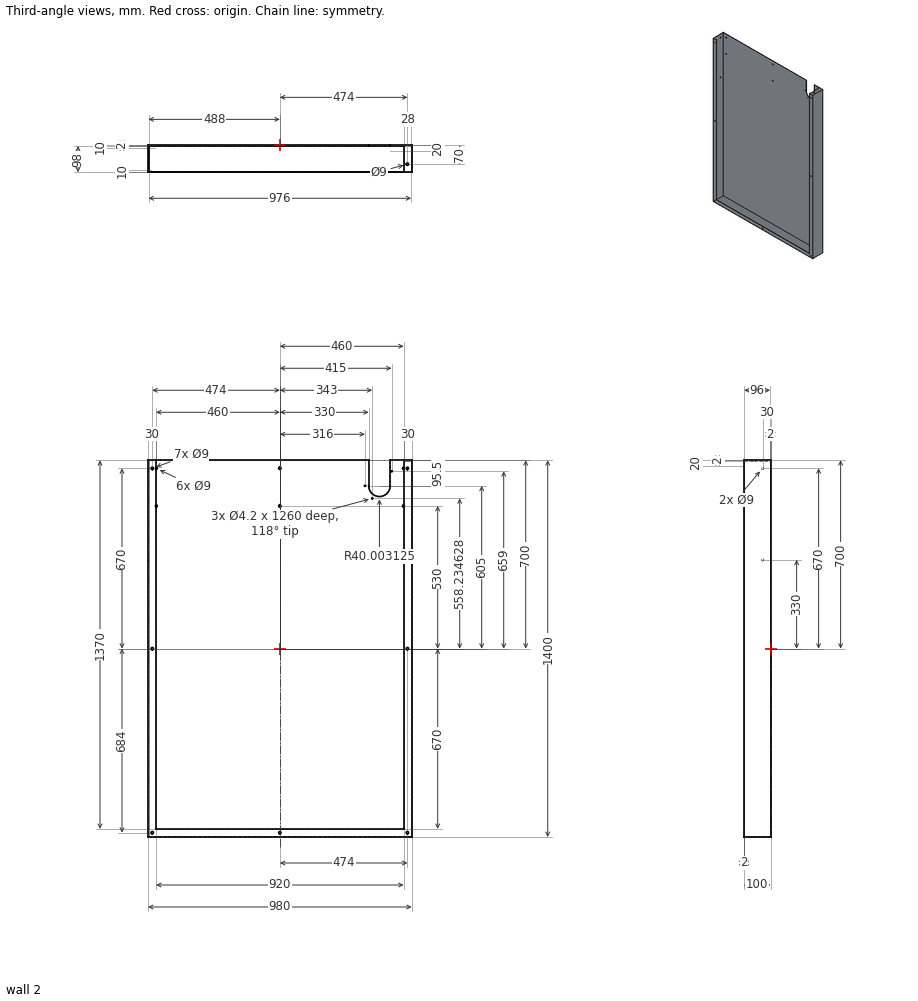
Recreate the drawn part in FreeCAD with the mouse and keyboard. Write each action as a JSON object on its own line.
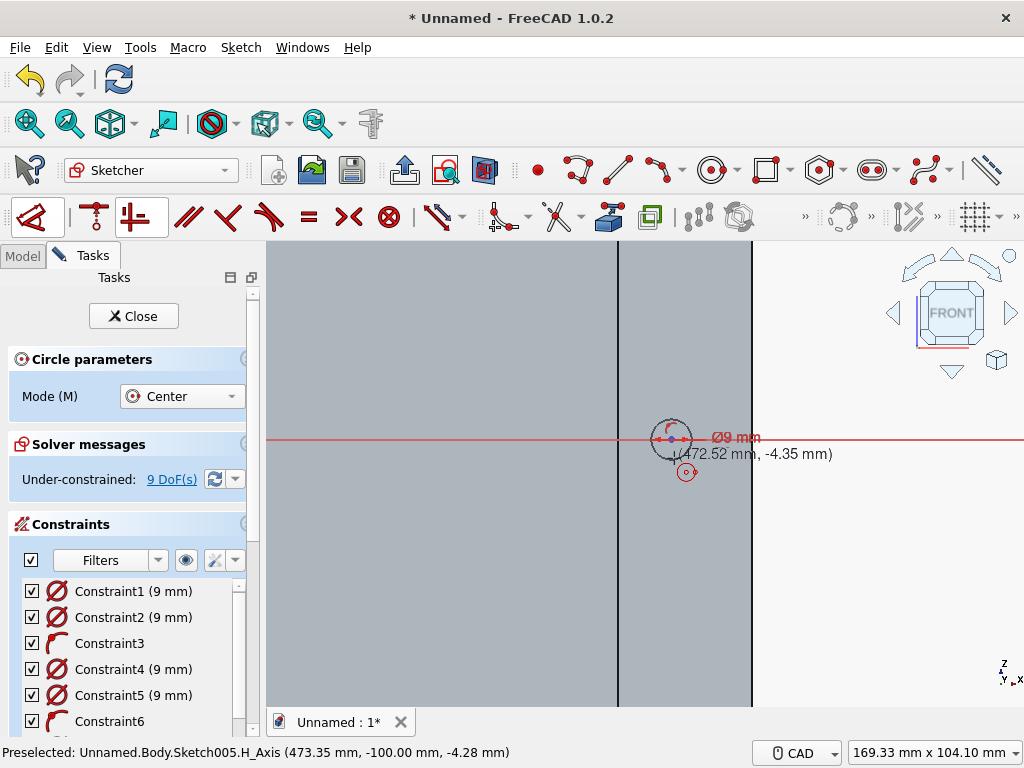
{"action": "scroll", "coordinate": [682, 474], "scroll_direction": "down", "scroll_amount": 15}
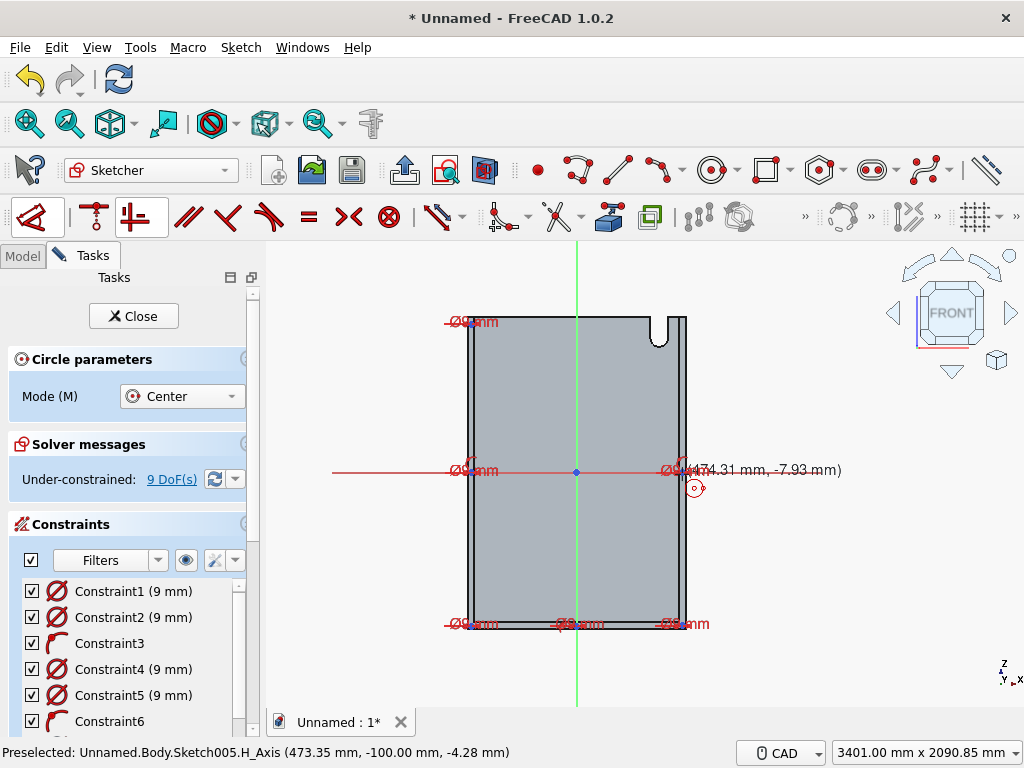
{"action": "scroll", "coordinate": [682, 323], "scroll_direction": "up", "scroll_amount": 16}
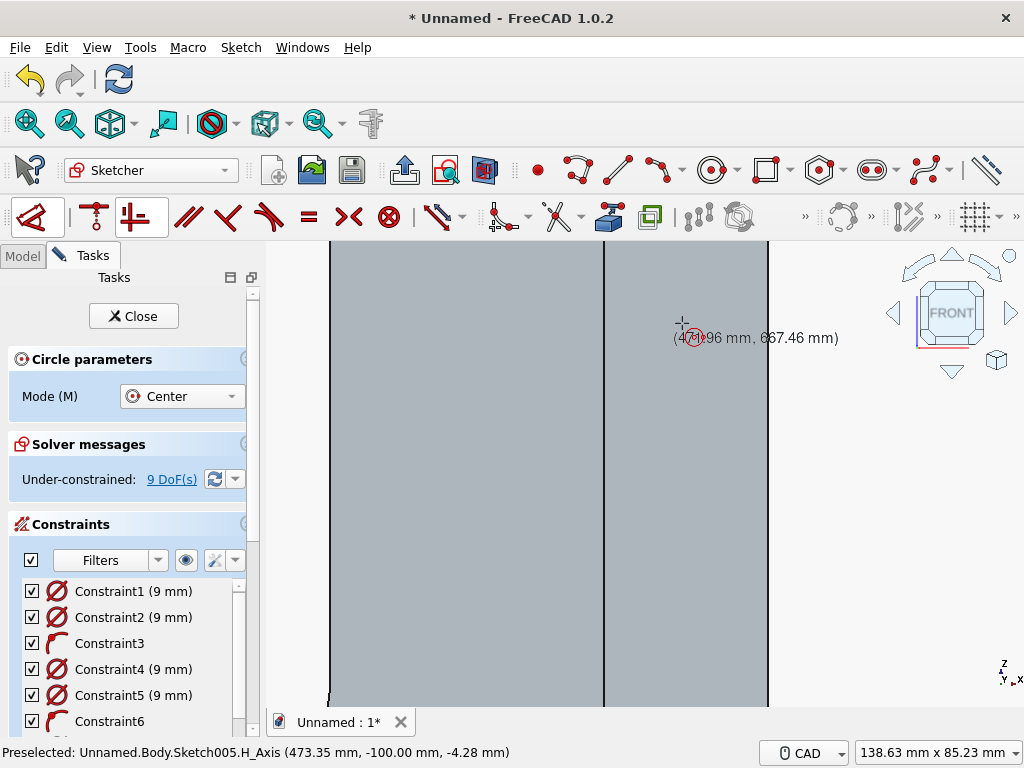
{"action": "scroll", "coordinate": [682, 323], "scroll_direction": "down", "scroll_amount": 16}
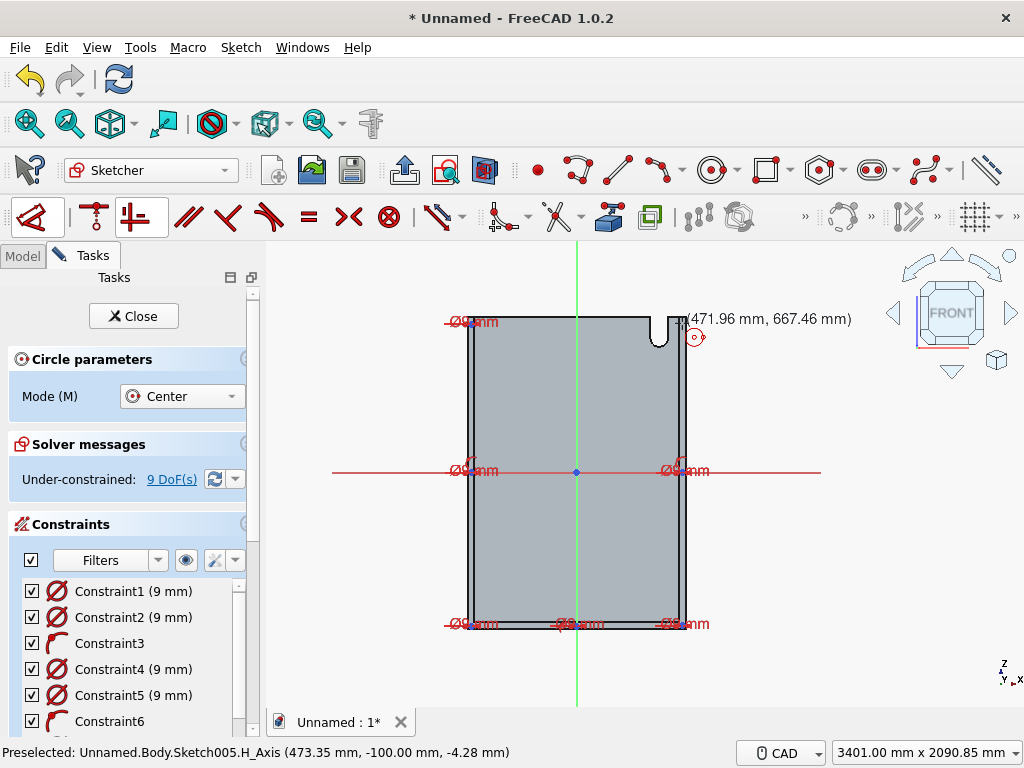
{"action": "left_click", "coordinate": [682, 323]}
{"action": "mouse_move", "coordinate": [683, 323]}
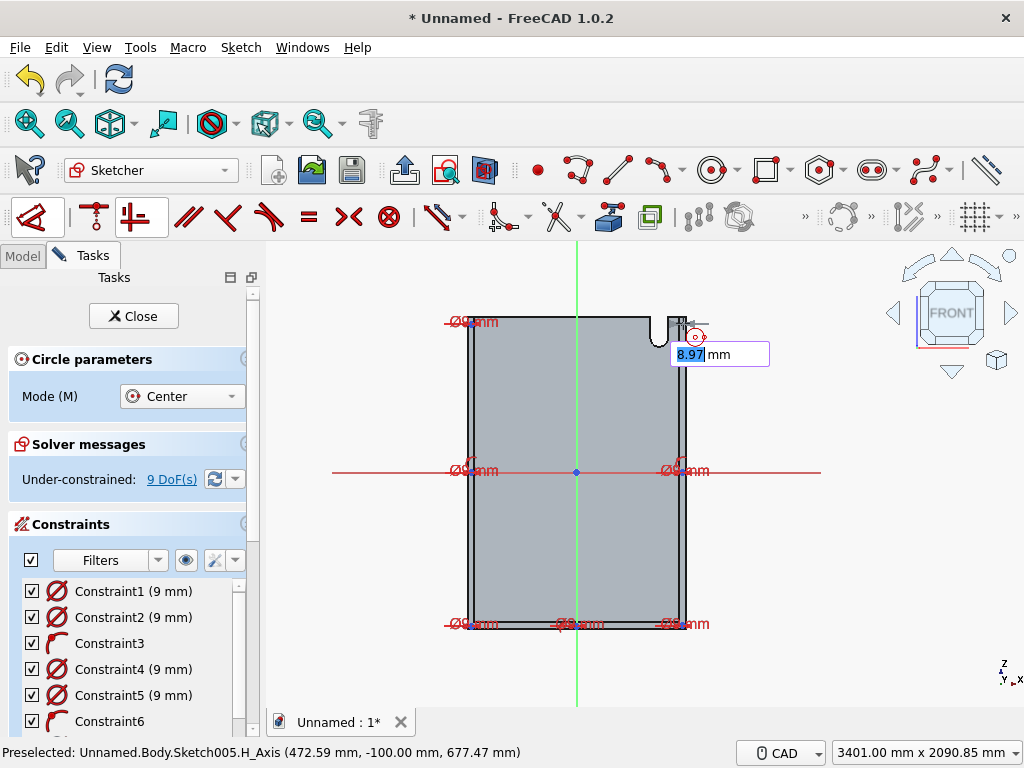
{"action": "type", "text": "9"}
{"action": "key", "text": "Return"}
{"action": "key", "text": "Escape"}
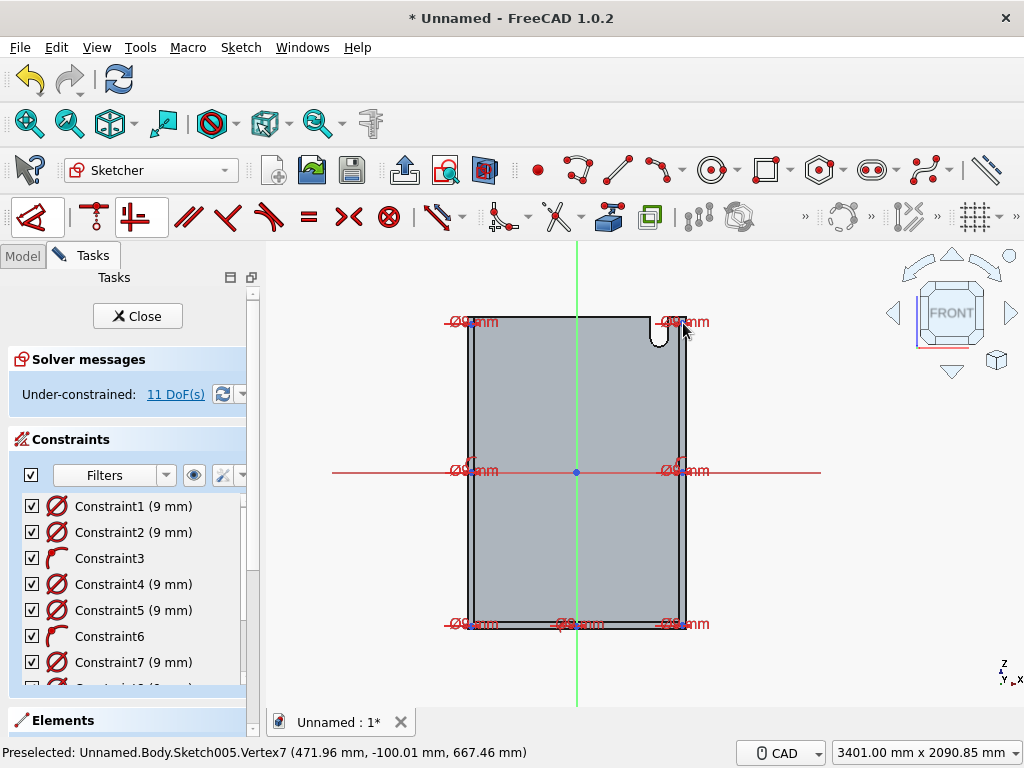
{"action": "left_click", "coordinate": [471, 626]}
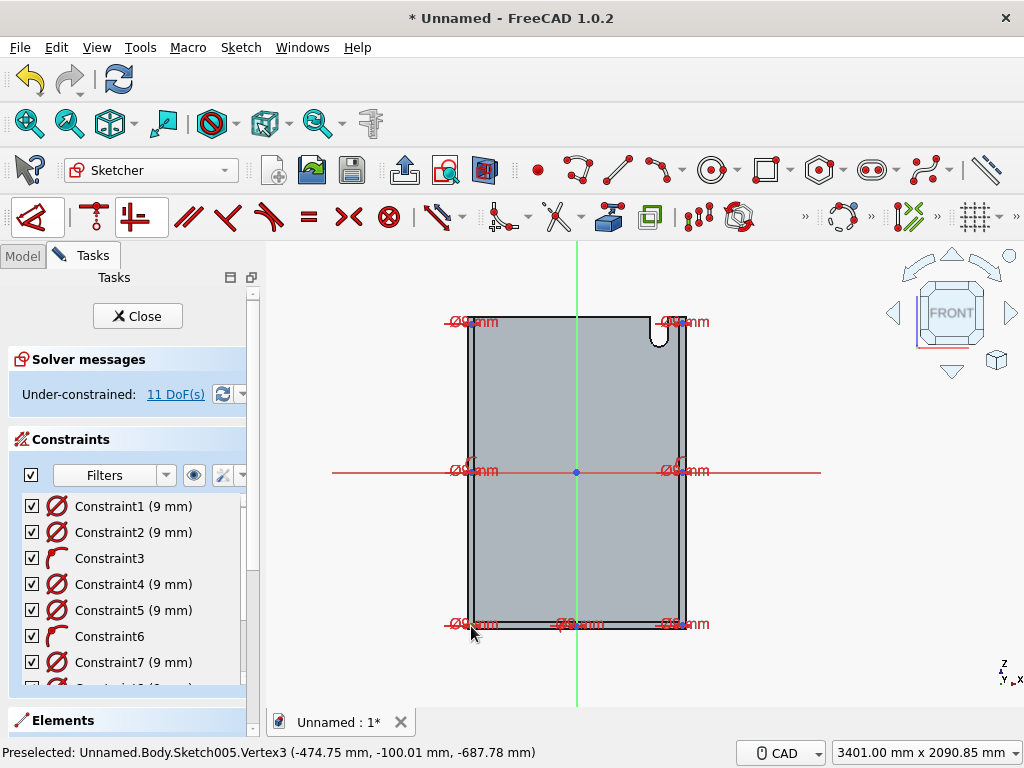
{"action": "left_click", "coordinate": [682, 626]}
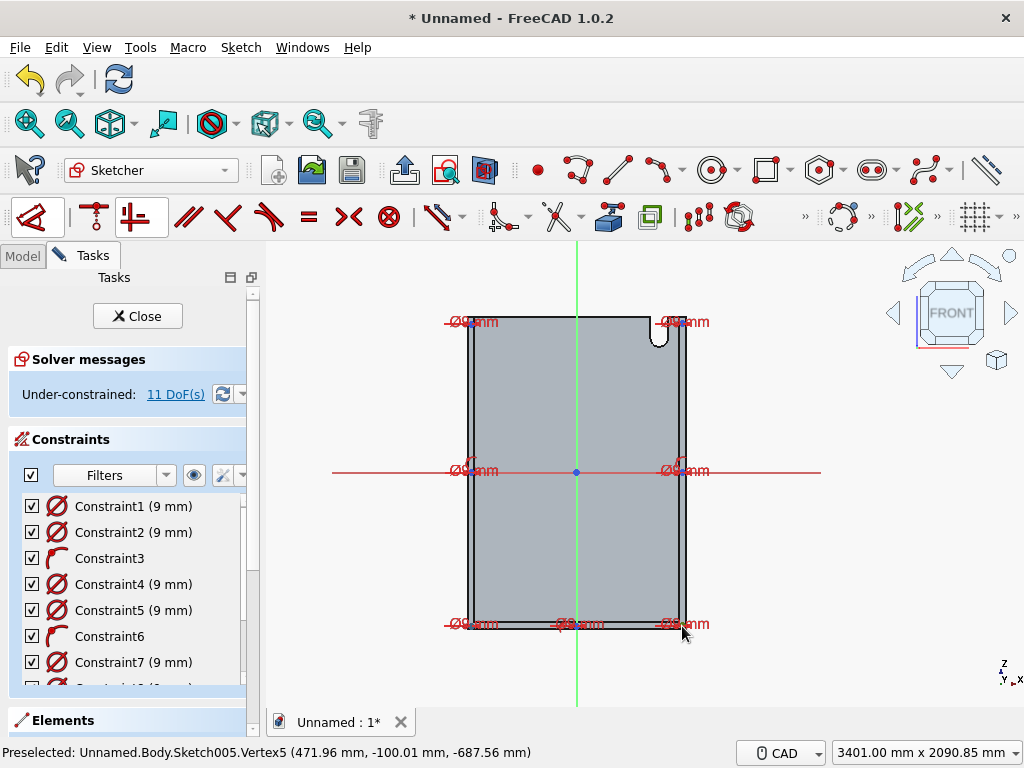
{"action": "left_click", "coordinate": [577, 591]}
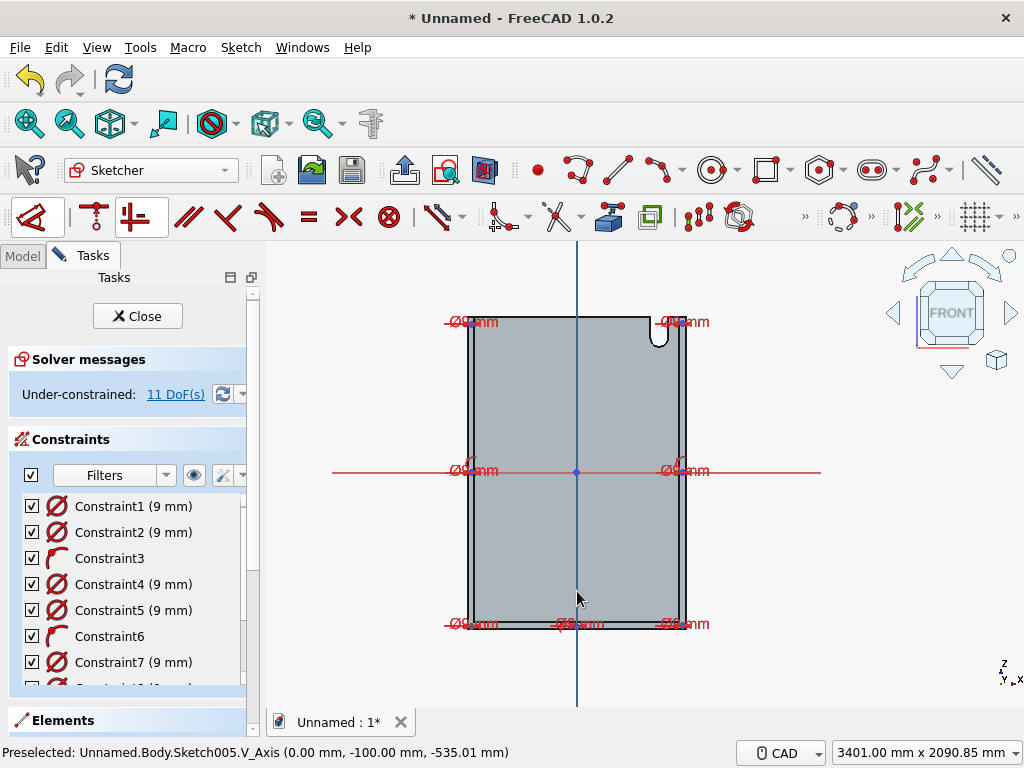
{"action": "left_click", "coordinate": [350, 218]}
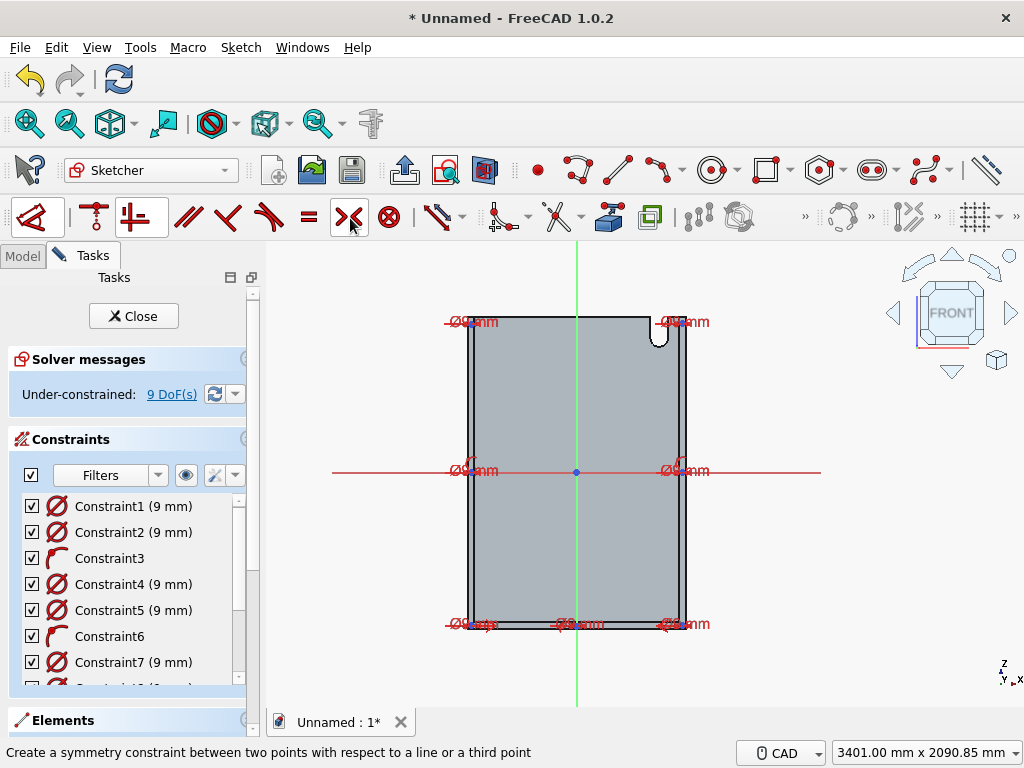
{"action": "left_click", "coordinate": [471, 324]}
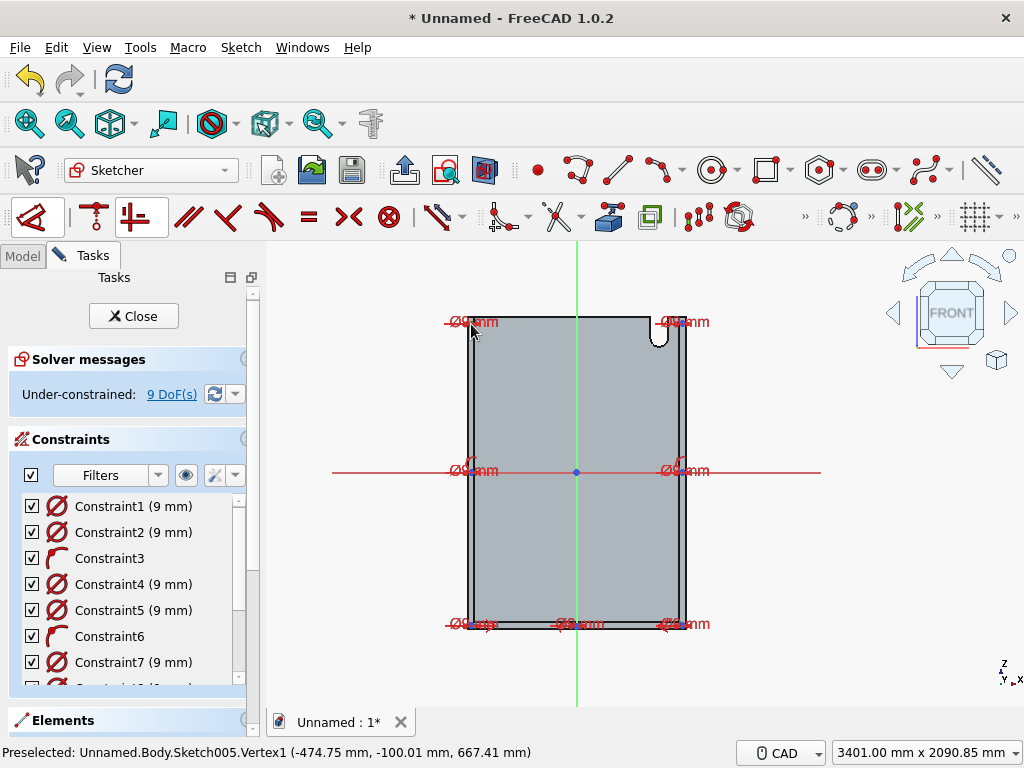
{"action": "left_click", "coordinate": [682, 324]}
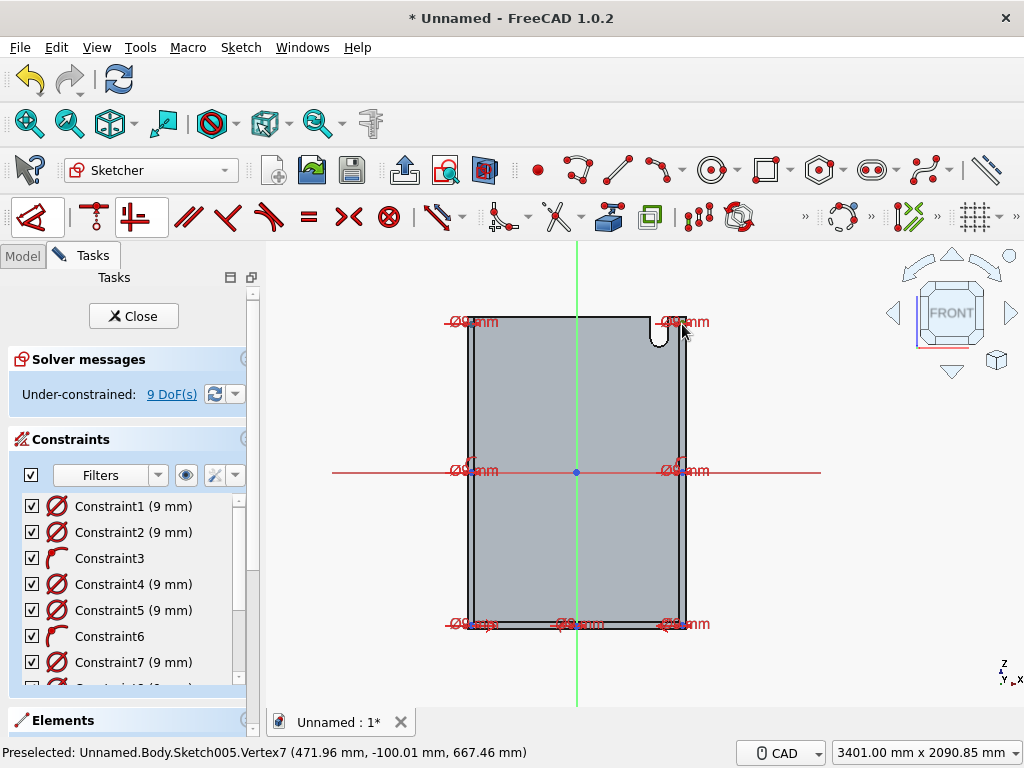
{"action": "left_click", "coordinate": [577, 591]}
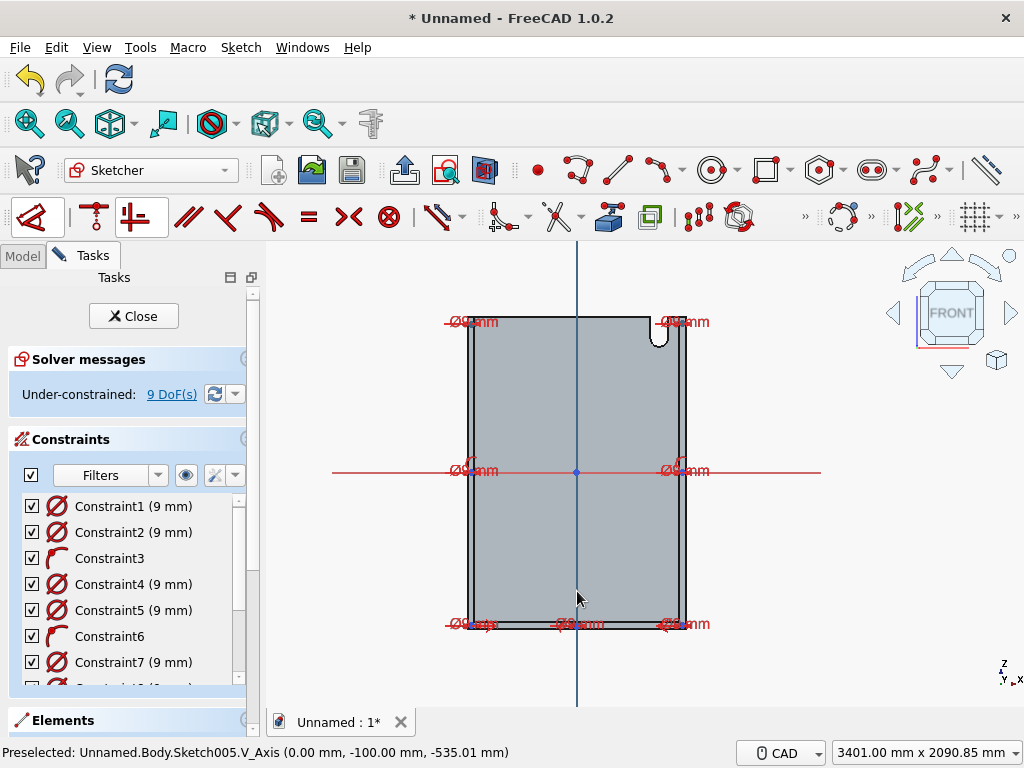
{"action": "left_click", "coordinate": [350, 218]}